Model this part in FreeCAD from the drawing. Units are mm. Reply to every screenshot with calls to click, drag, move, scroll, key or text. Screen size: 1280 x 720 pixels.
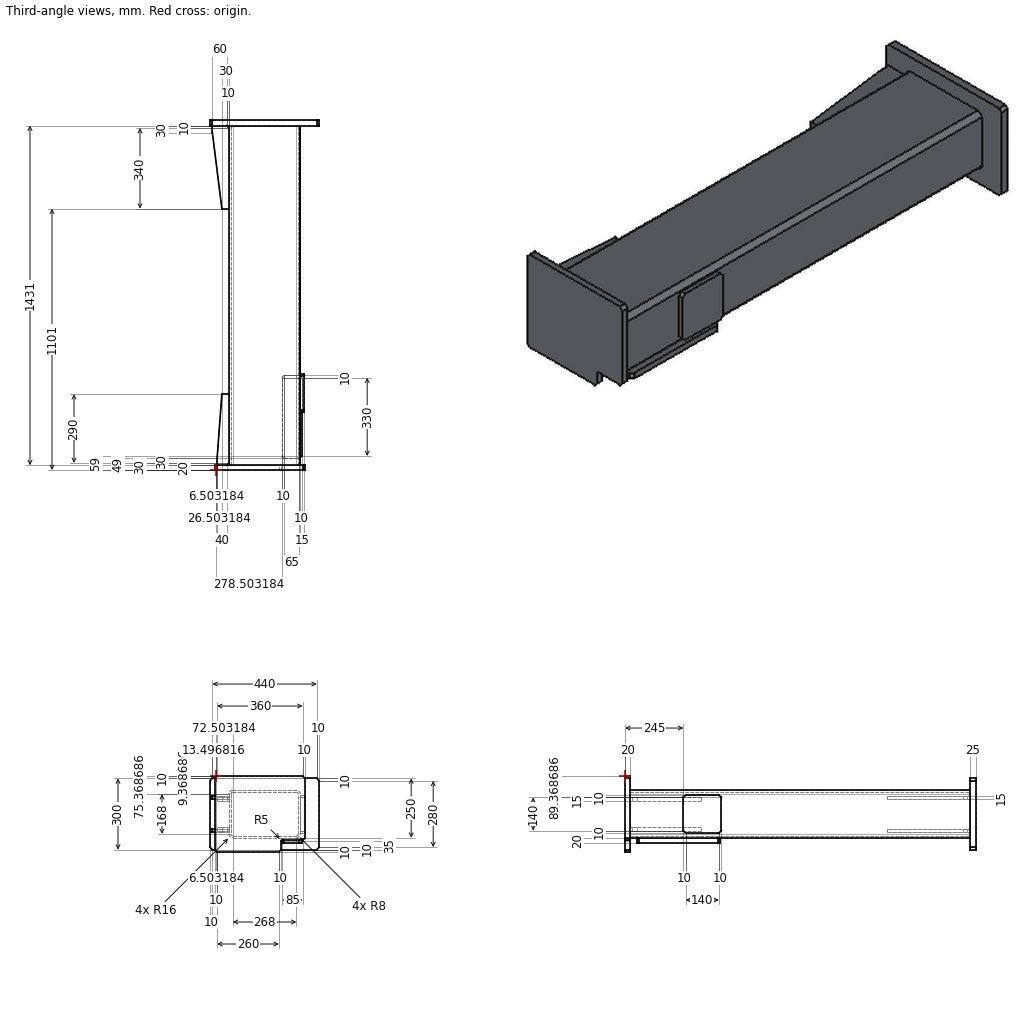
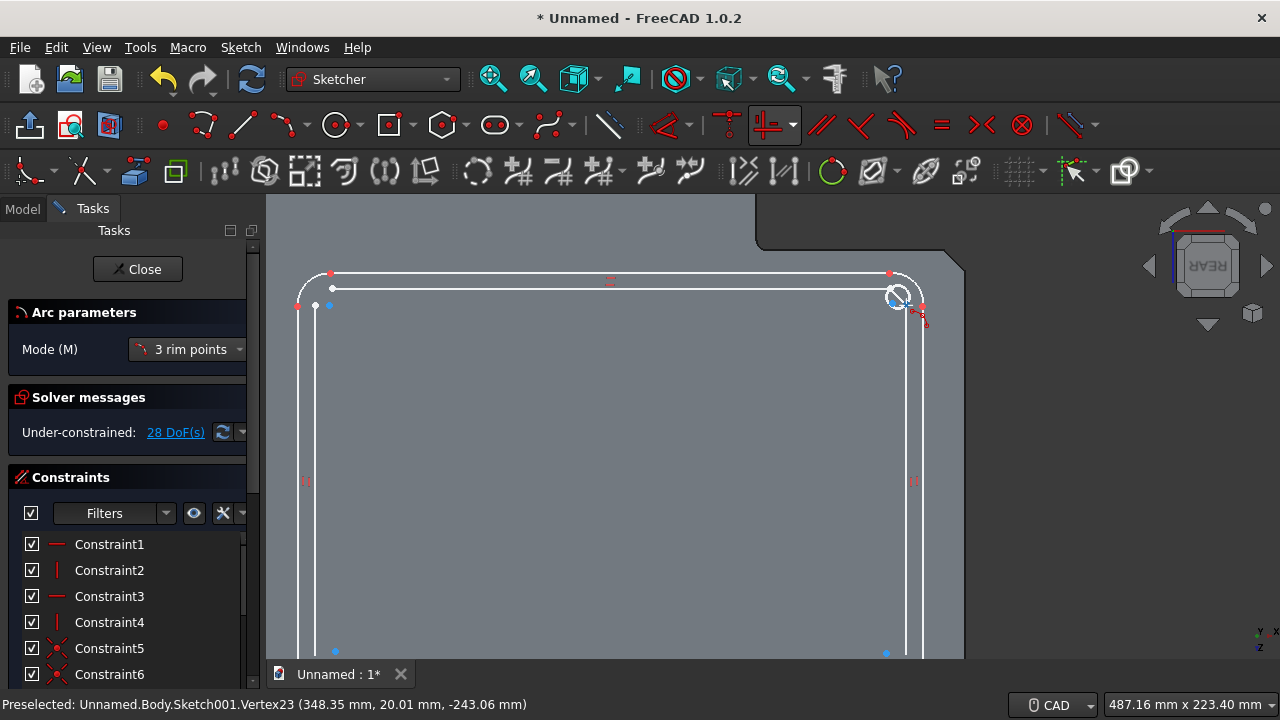
scroll(901, 293, up, 6)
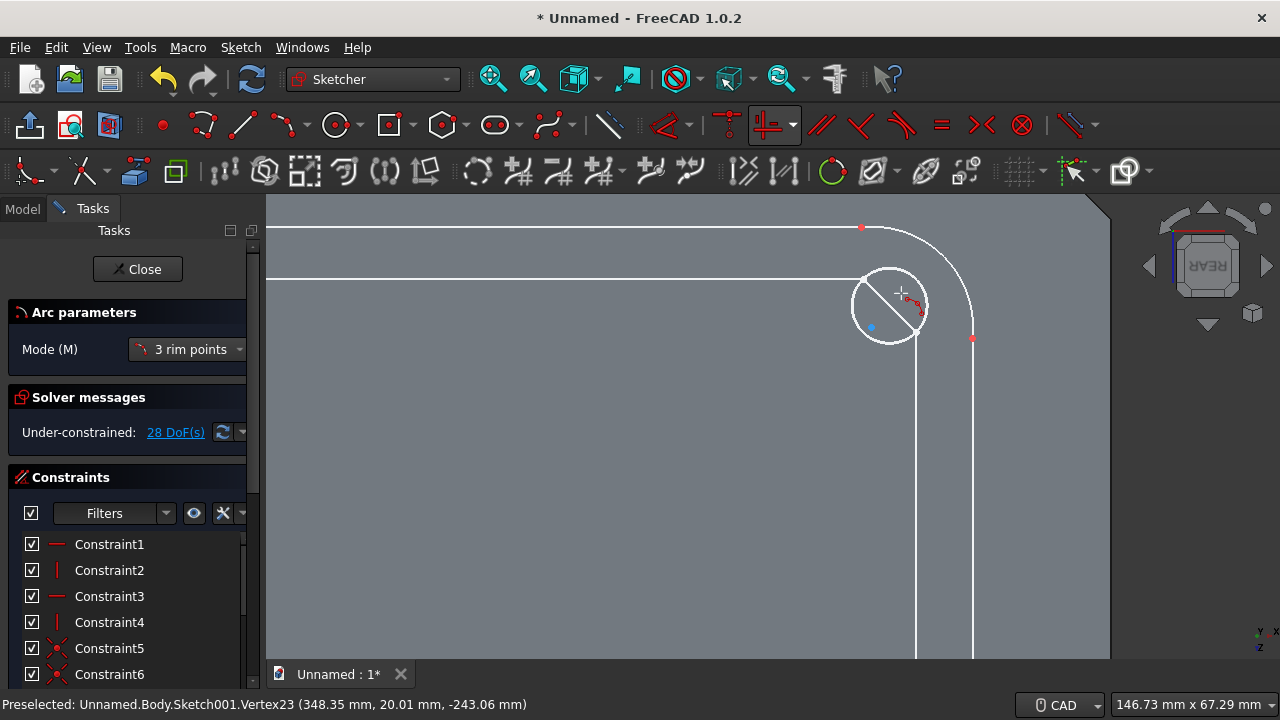
click(901, 291)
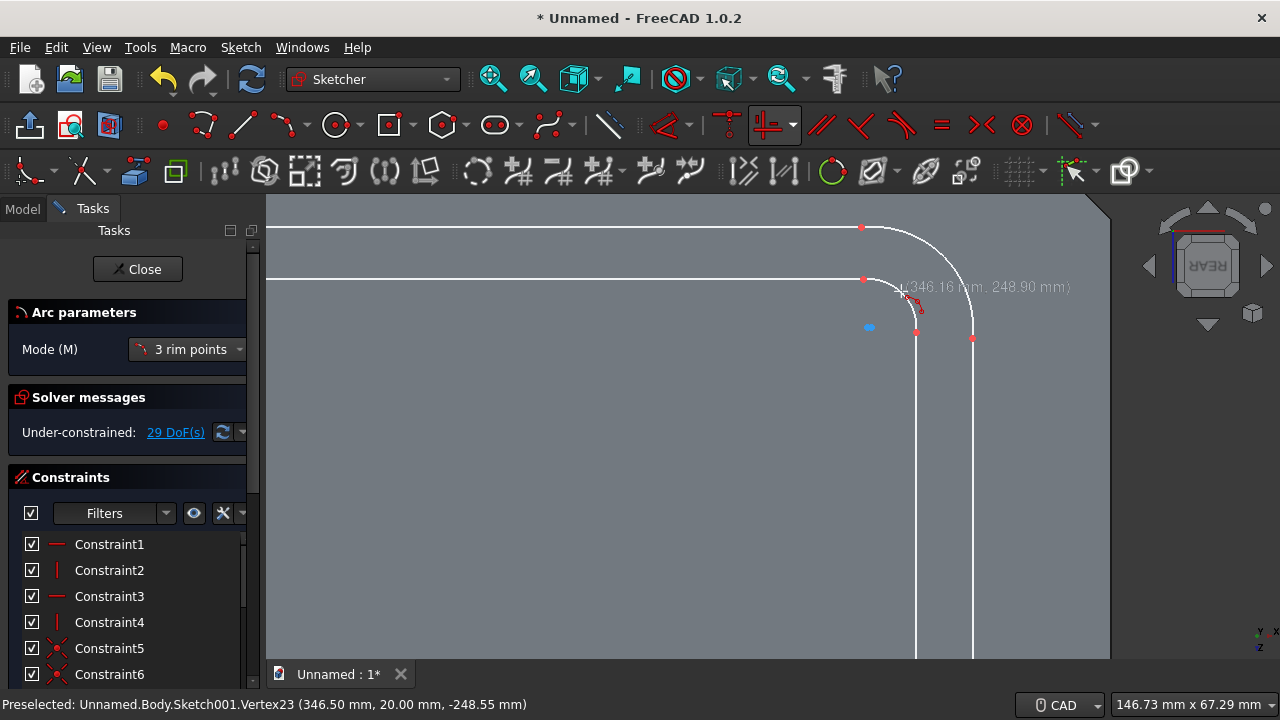
scroll(895, 290, down, 9)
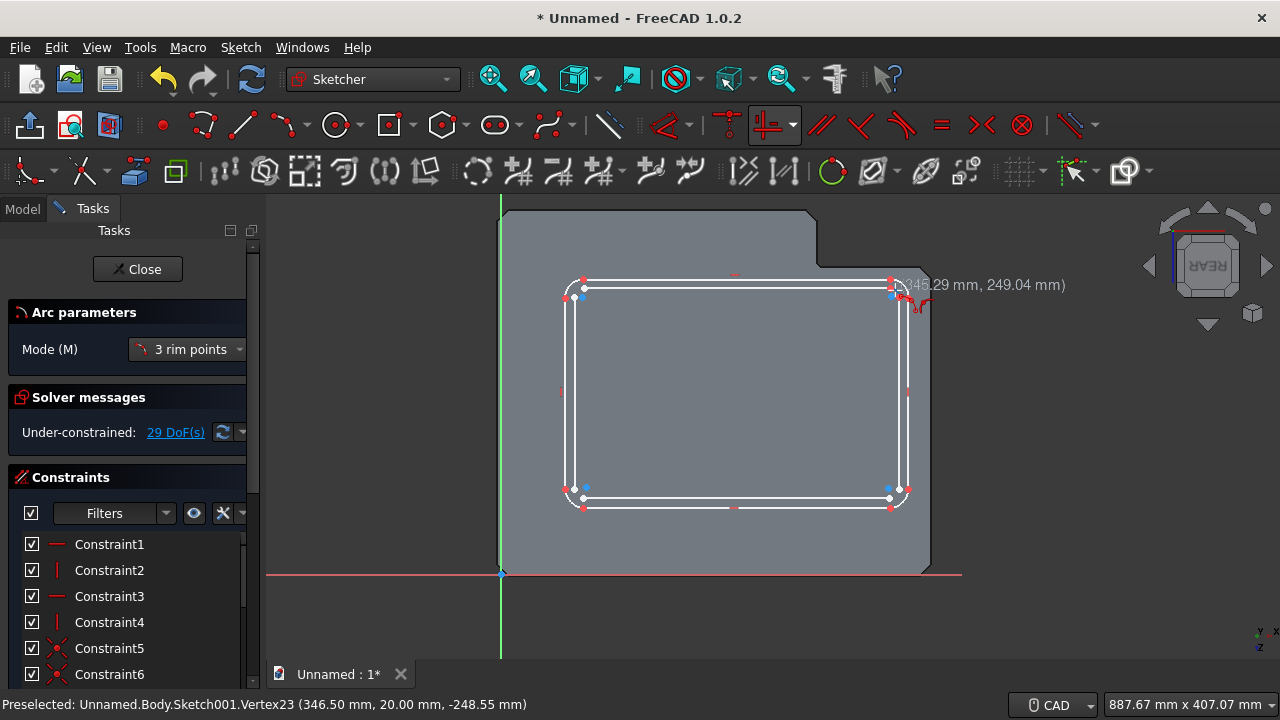
scroll(899, 489, up, 3)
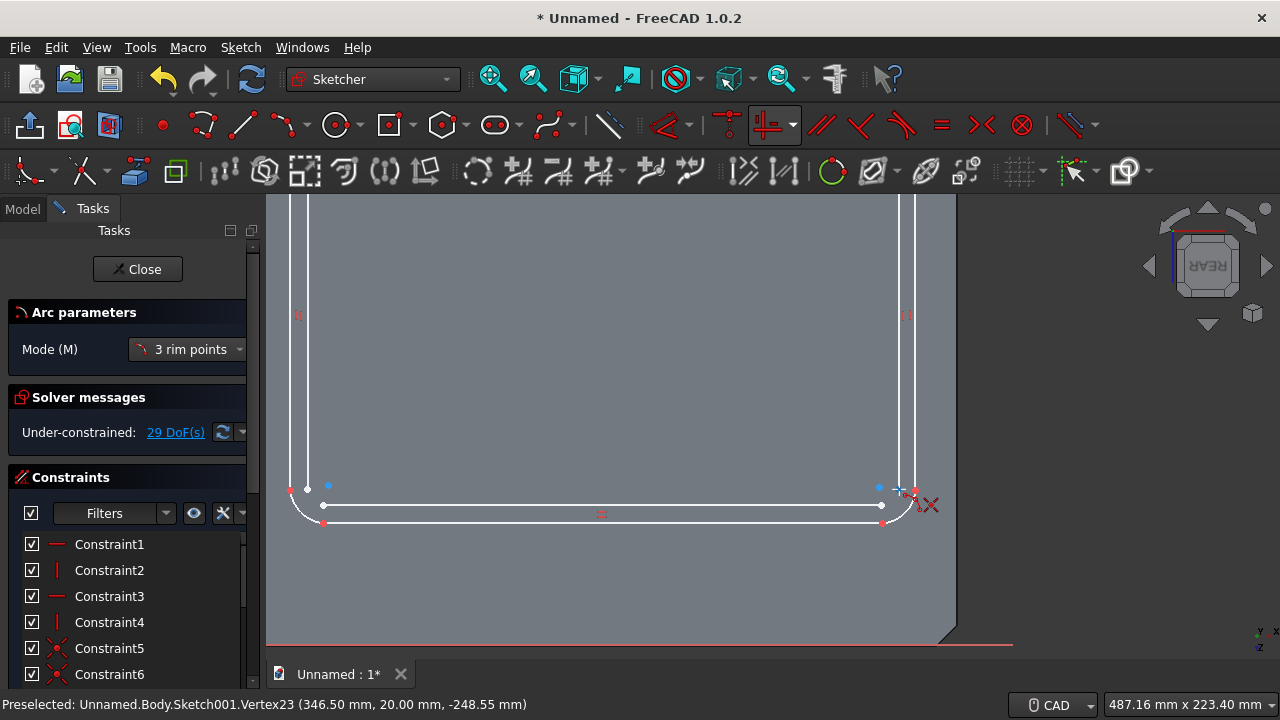
click(899, 489)
click(882, 505)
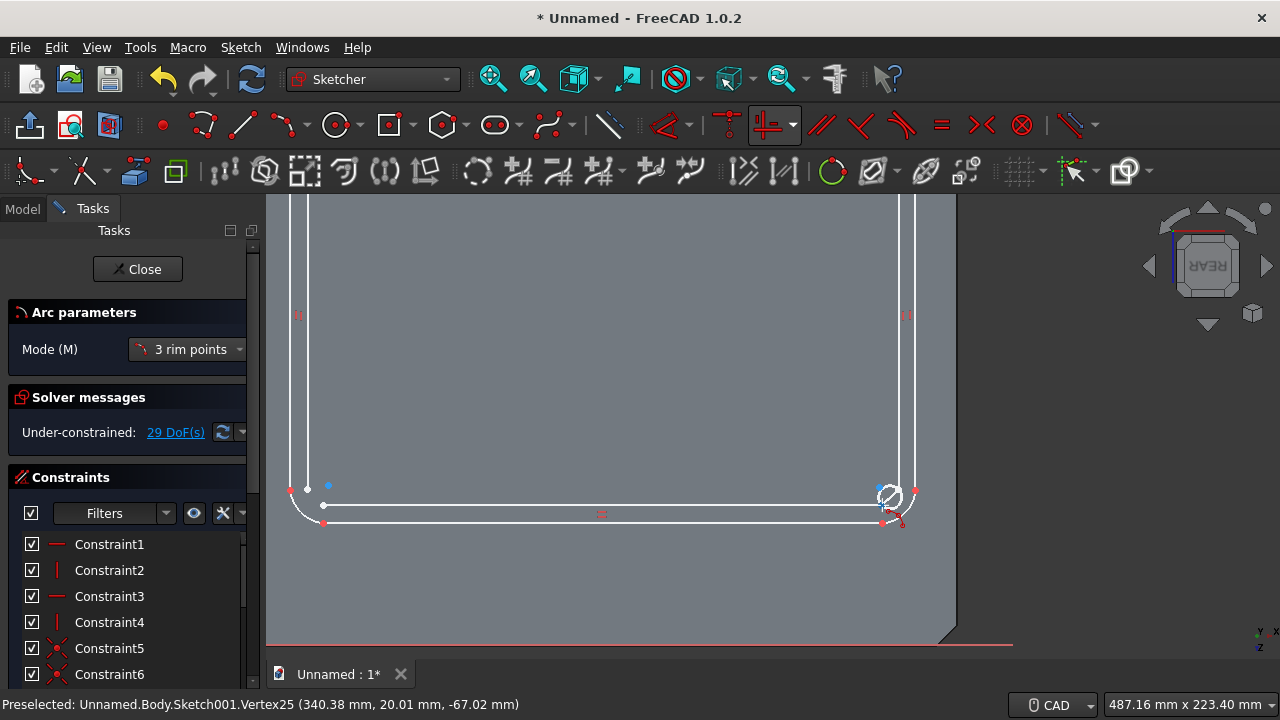
scroll(894, 500, up, 6)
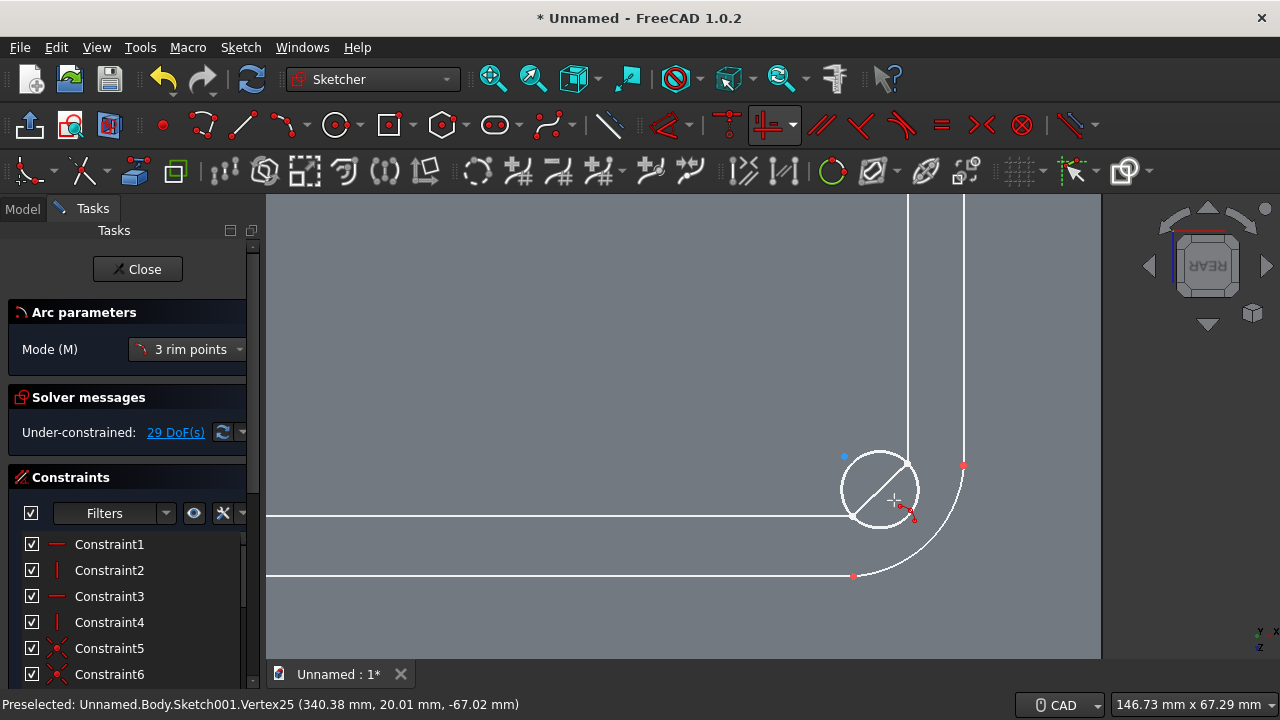
click(892, 498)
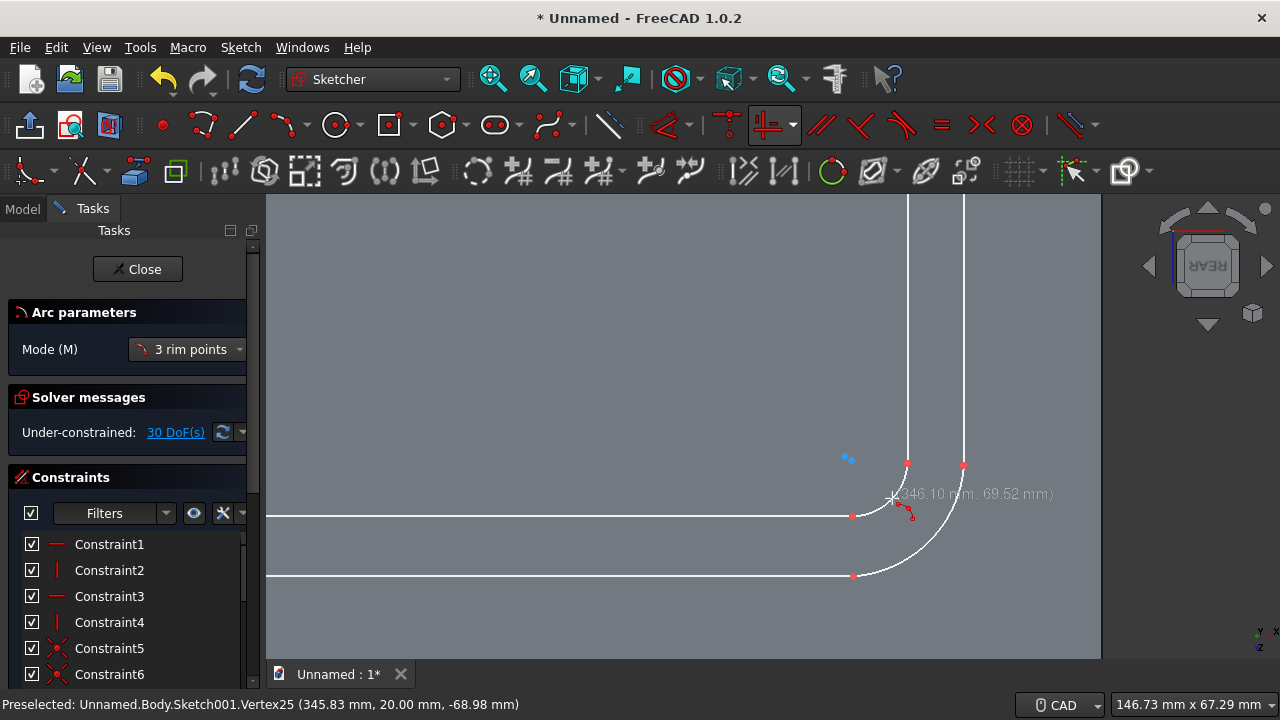
scroll(897, 494, down, 9)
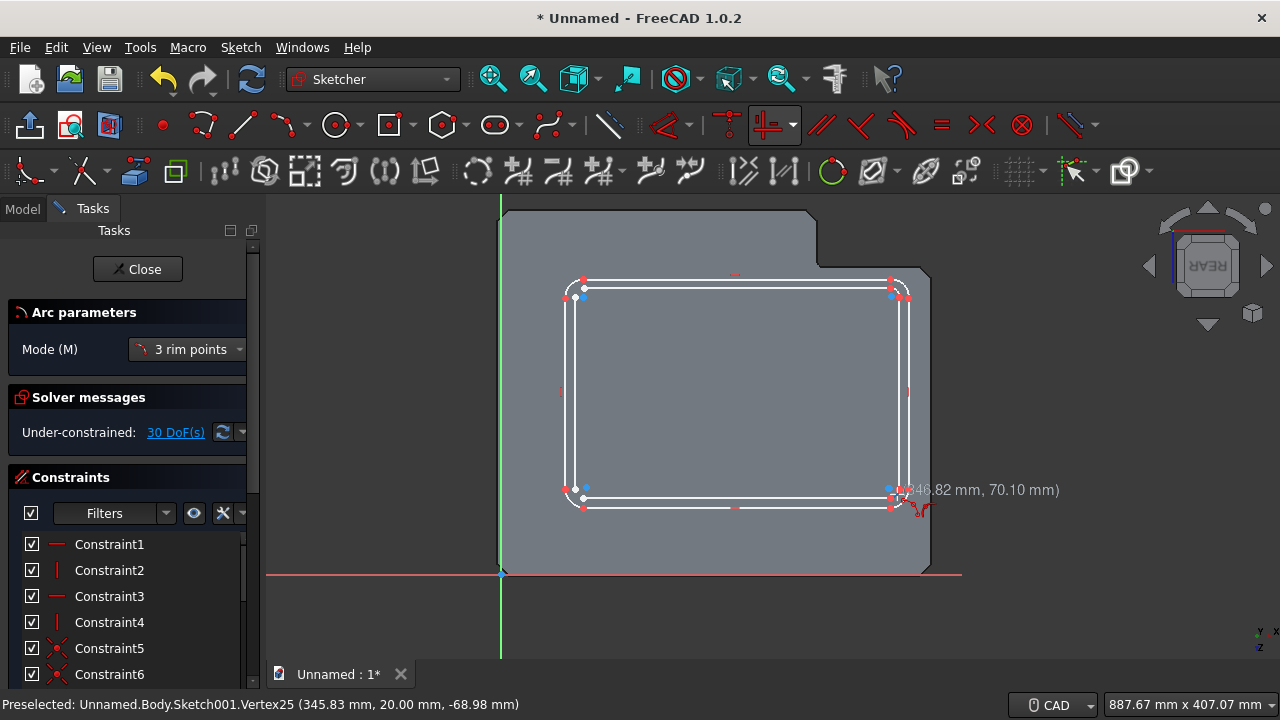
scroll(584, 498, up, 3)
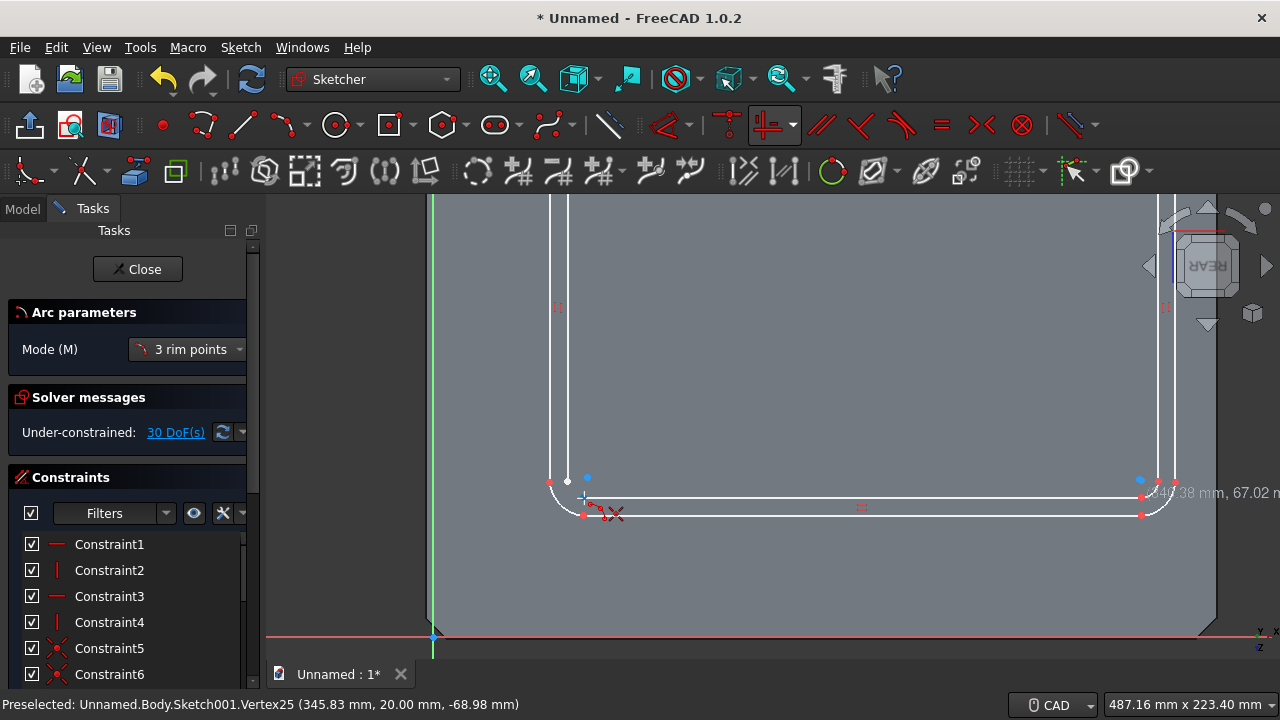
click(584, 498)
click(568, 482)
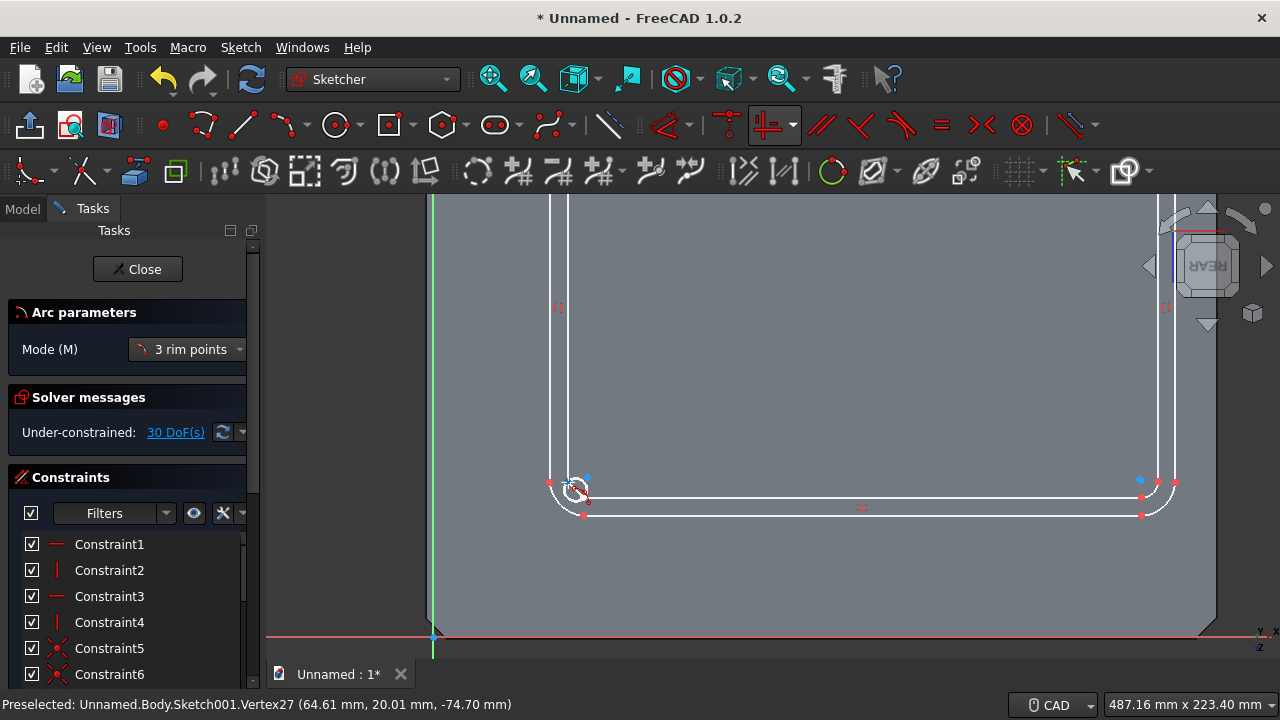
scroll(572, 492, up, 6)